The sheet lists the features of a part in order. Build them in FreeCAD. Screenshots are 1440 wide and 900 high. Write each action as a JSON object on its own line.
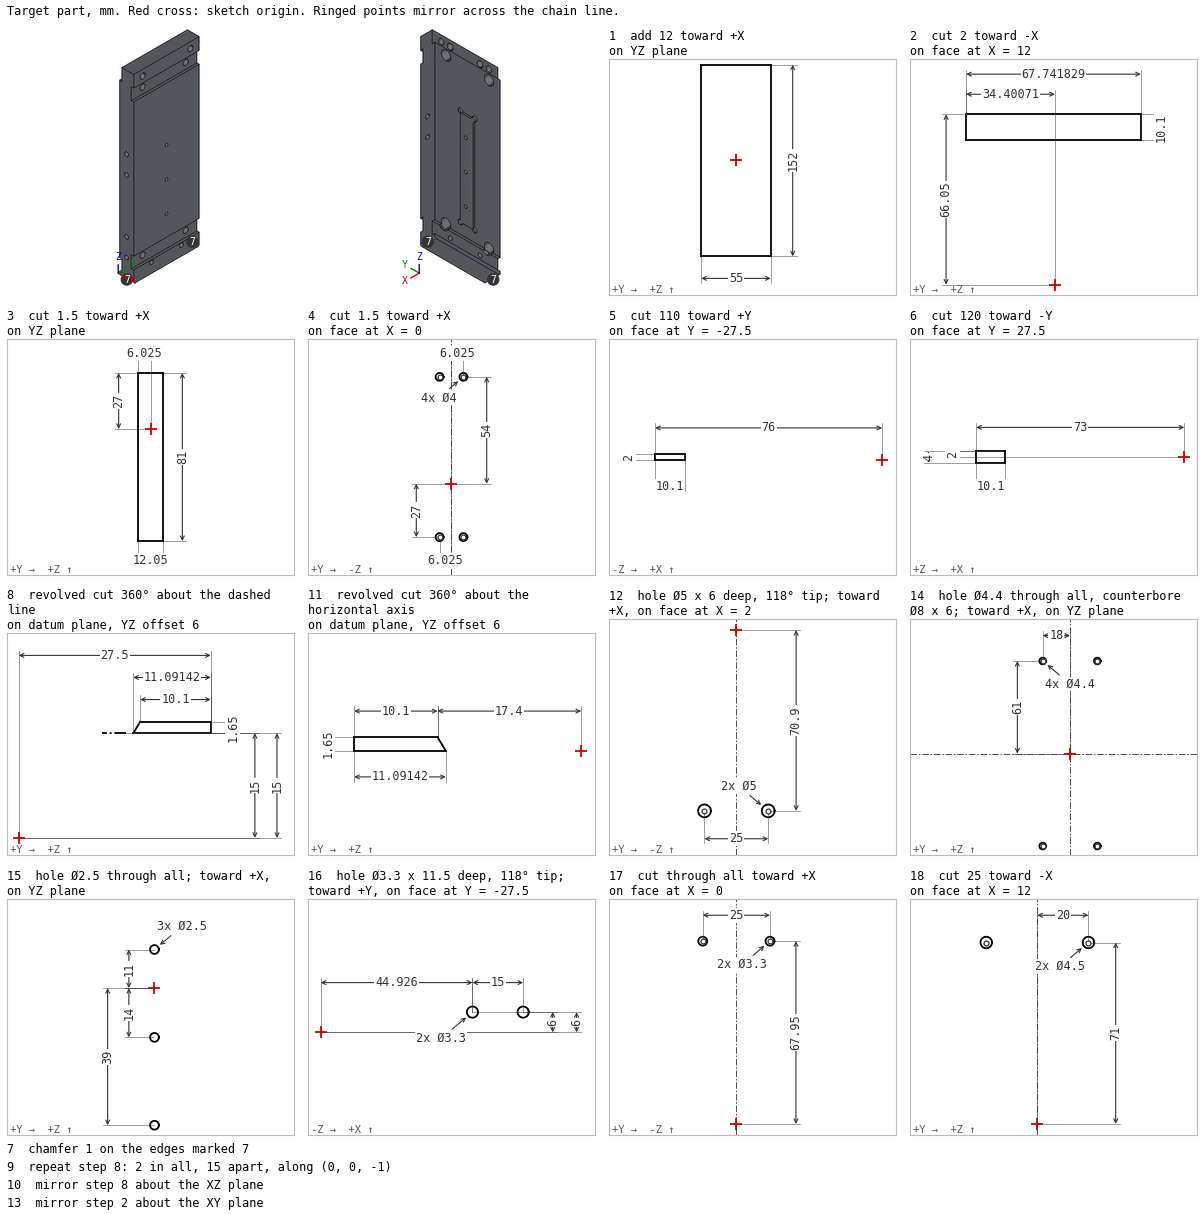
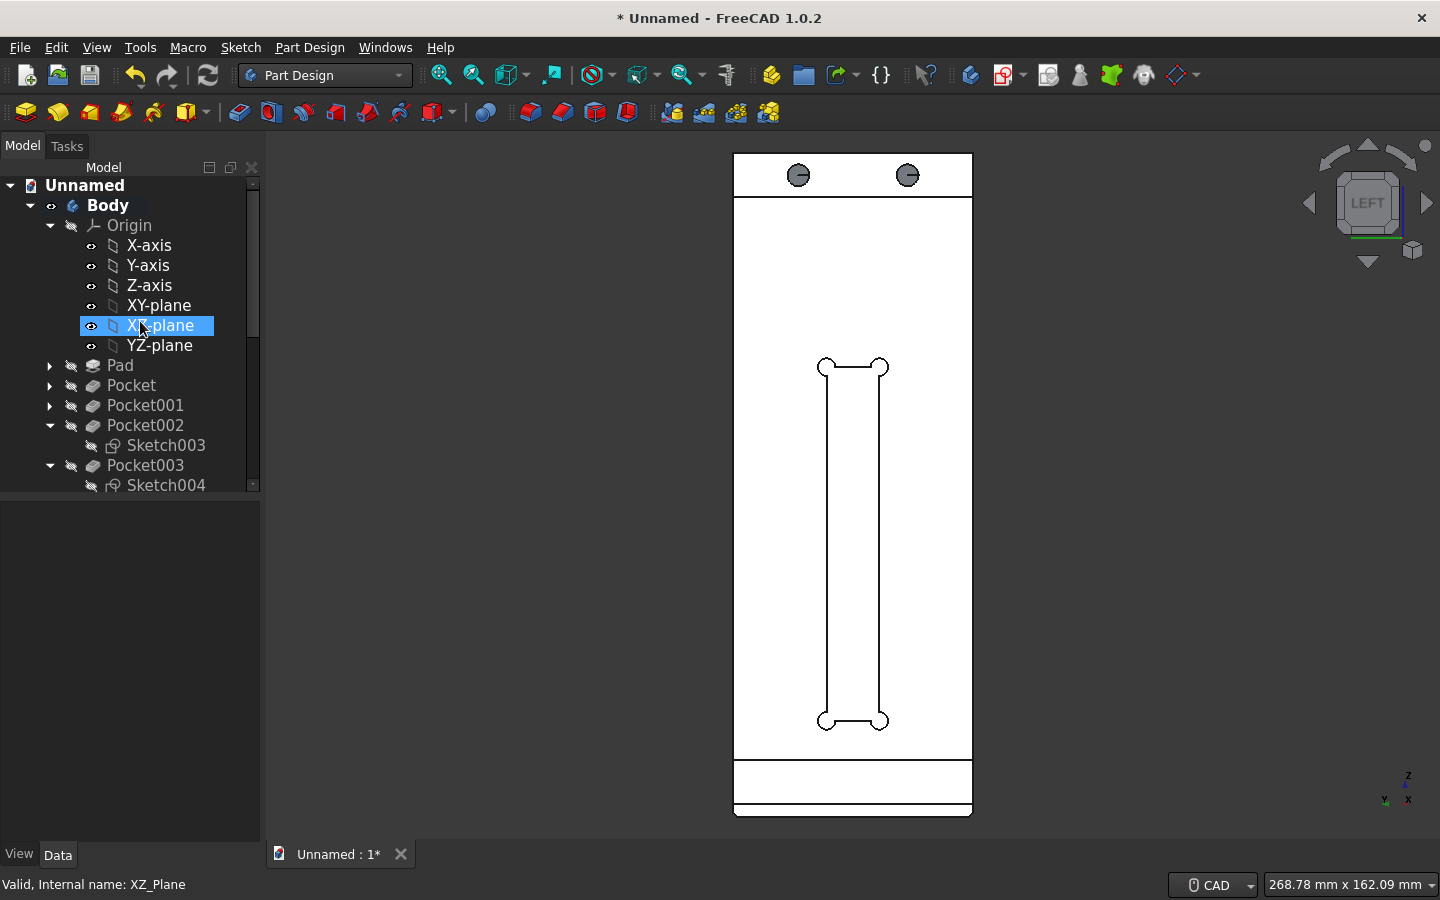
{"action": "left_click", "coordinate": [116, 386]}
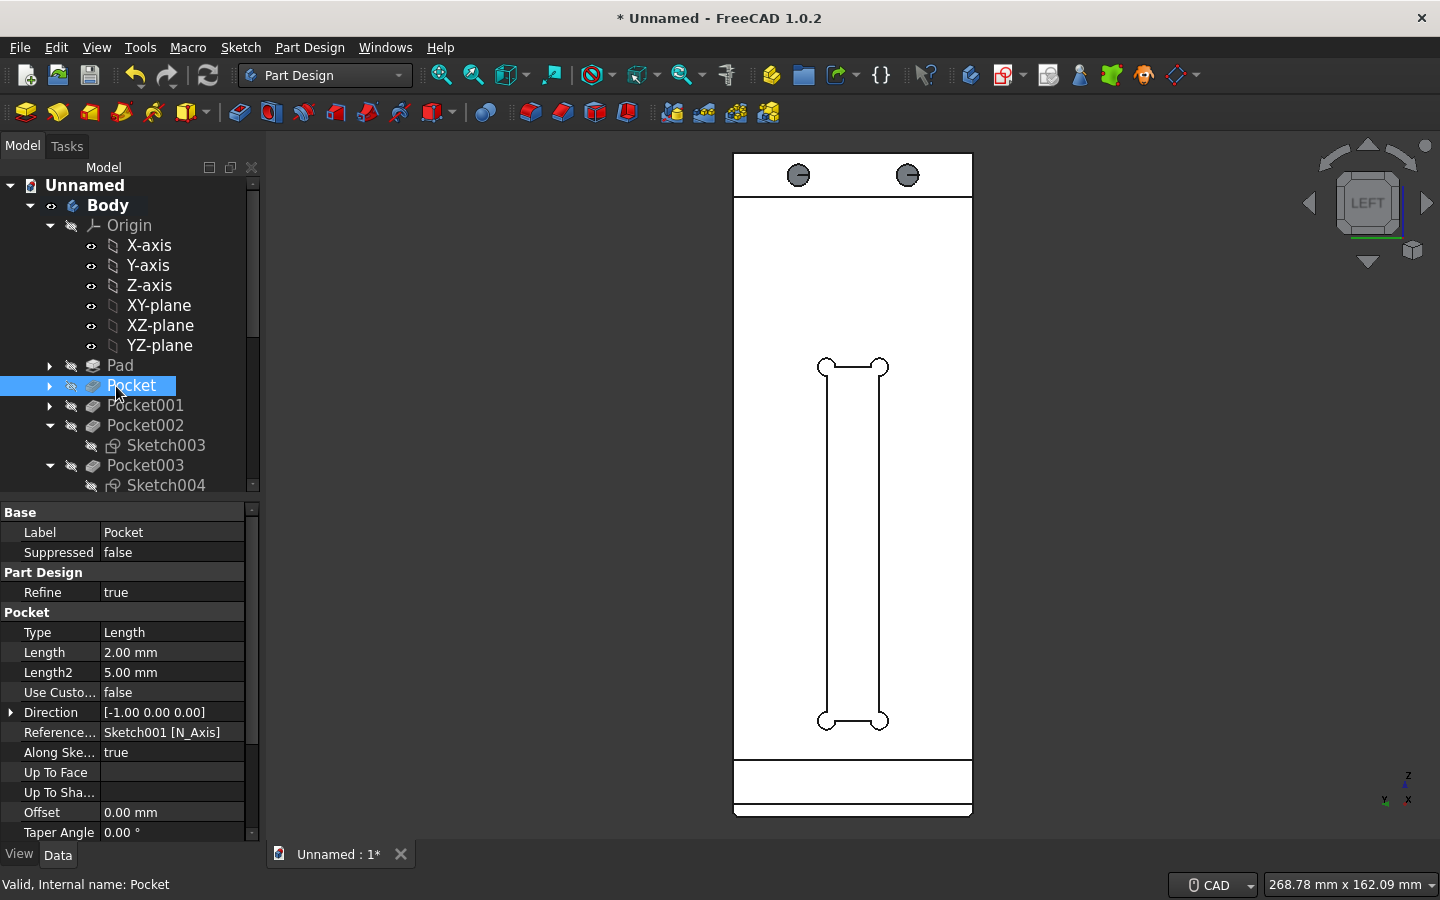
{"action": "left_click", "coordinate": [672, 112]}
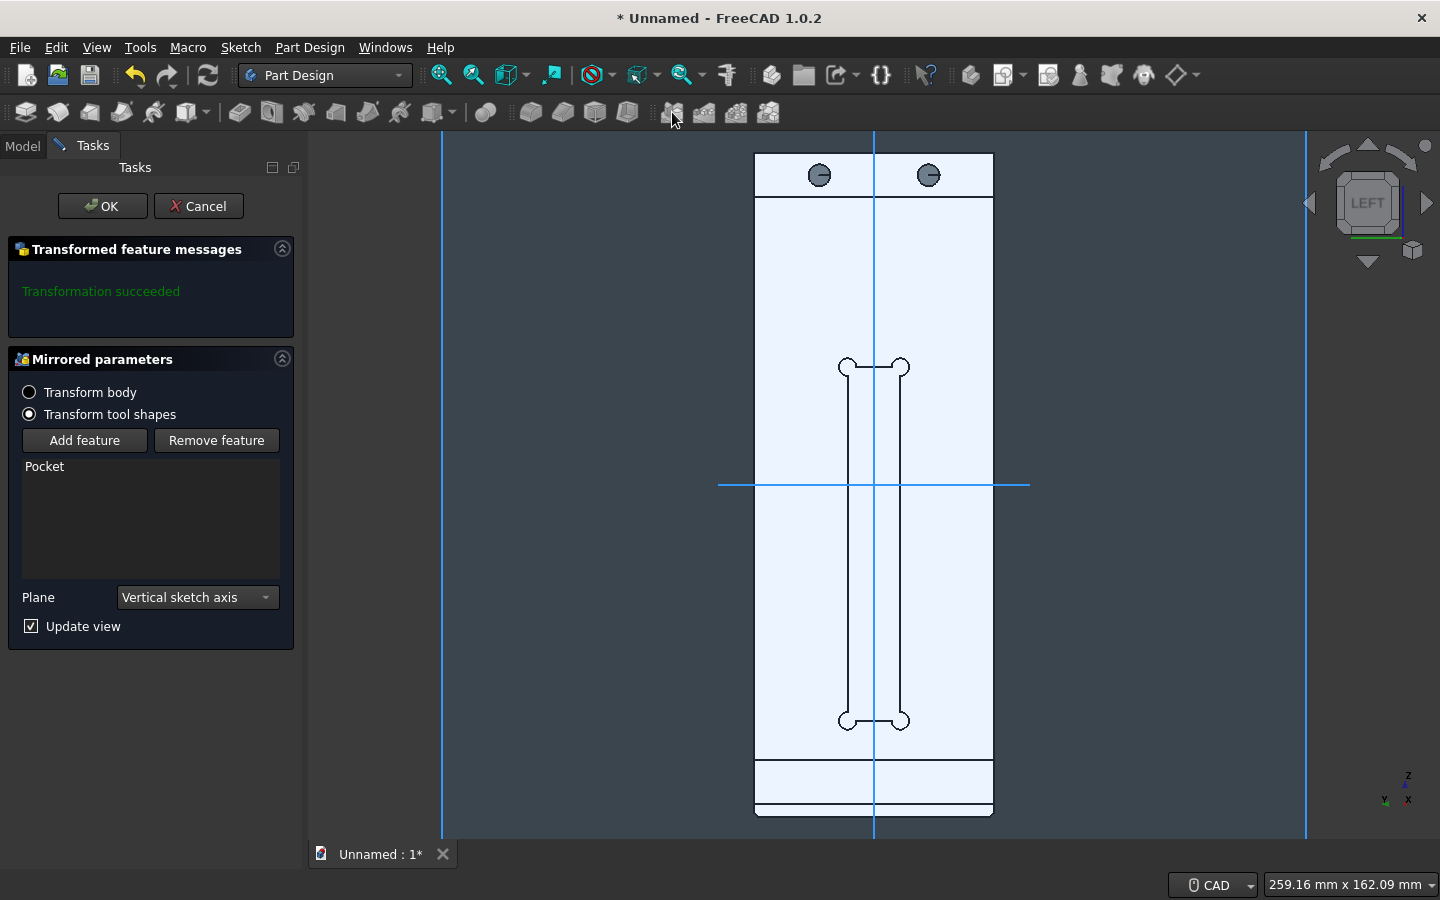
{"action": "left_click", "coordinate": [198, 598]}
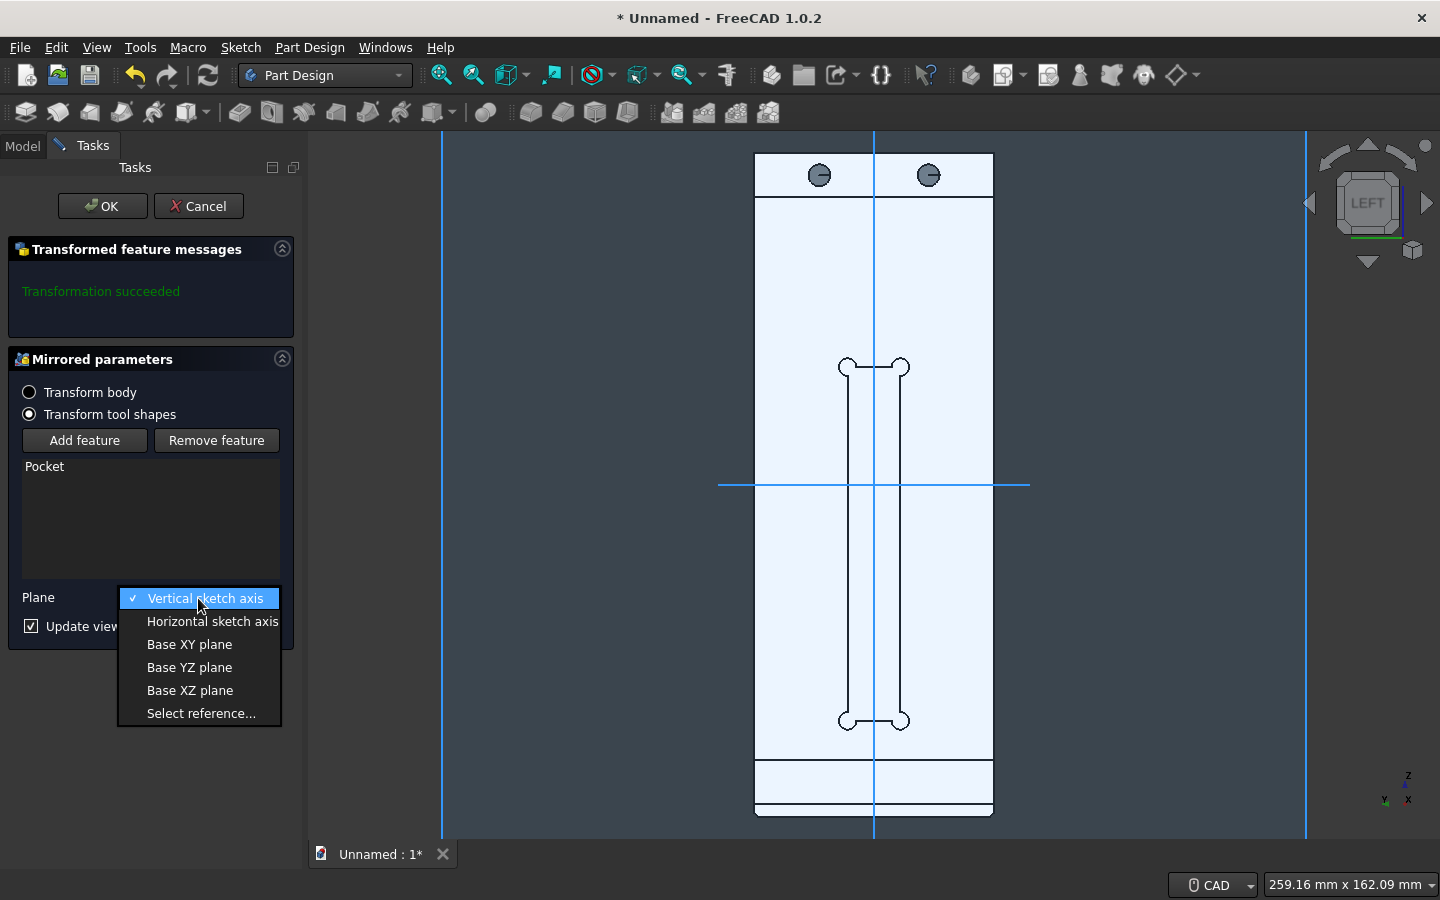
{"action": "left_click", "coordinate": [198, 644]}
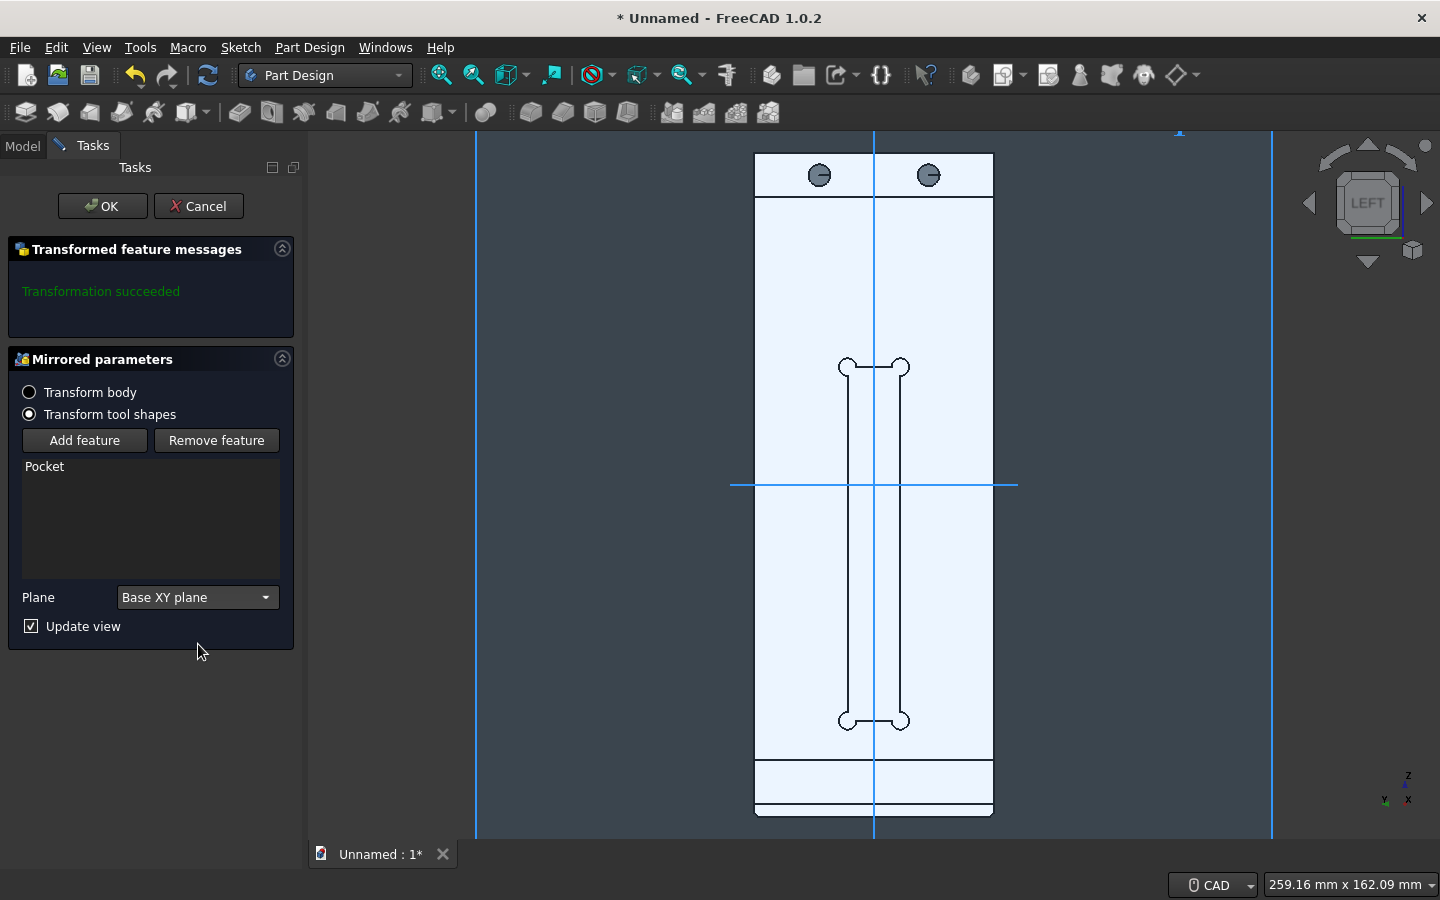
{"action": "left_click", "coordinate": [103, 206]}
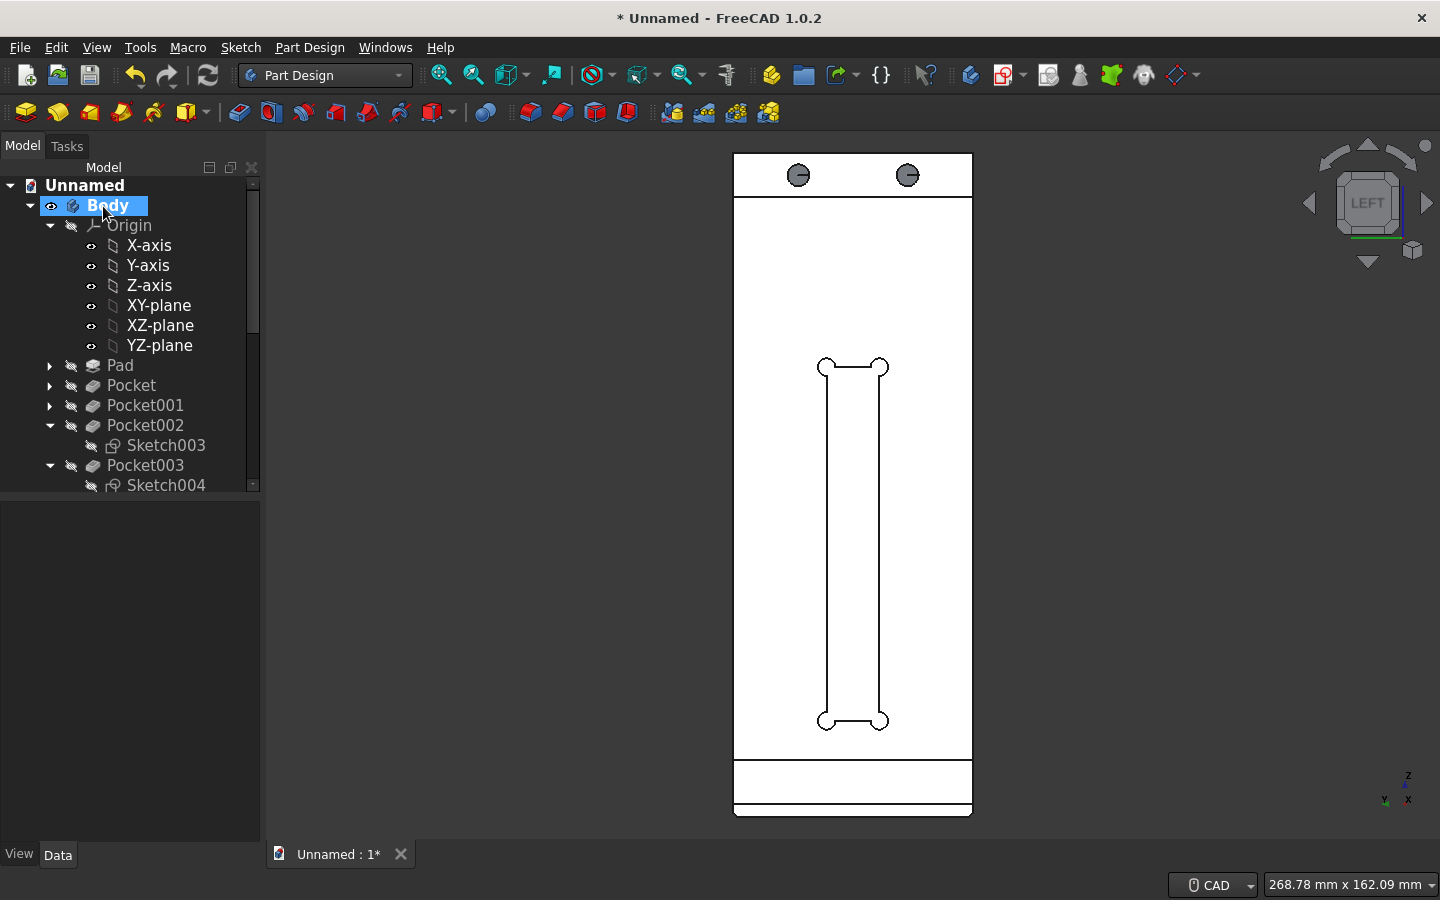
{"action": "left_click", "coordinate": [1004, 76]}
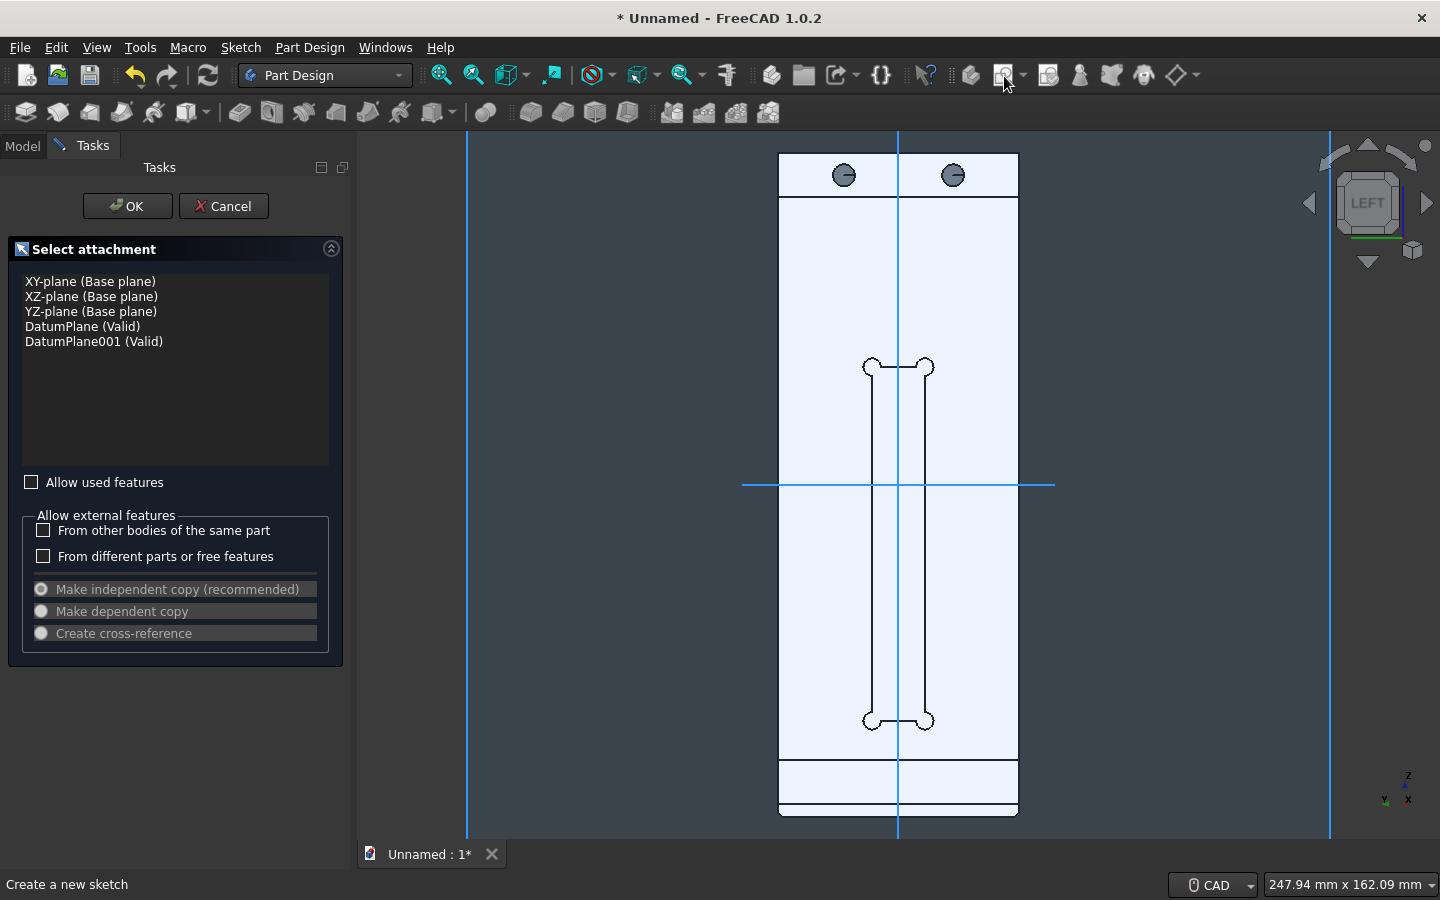
{"action": "left_click", "coordinate": [82, 312]}